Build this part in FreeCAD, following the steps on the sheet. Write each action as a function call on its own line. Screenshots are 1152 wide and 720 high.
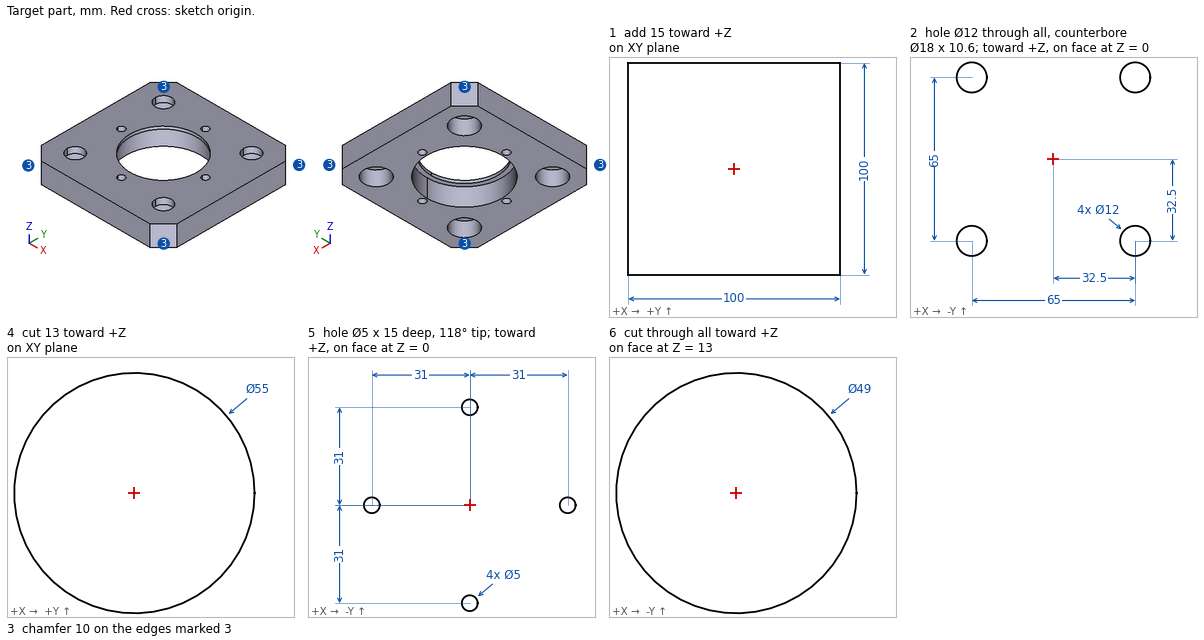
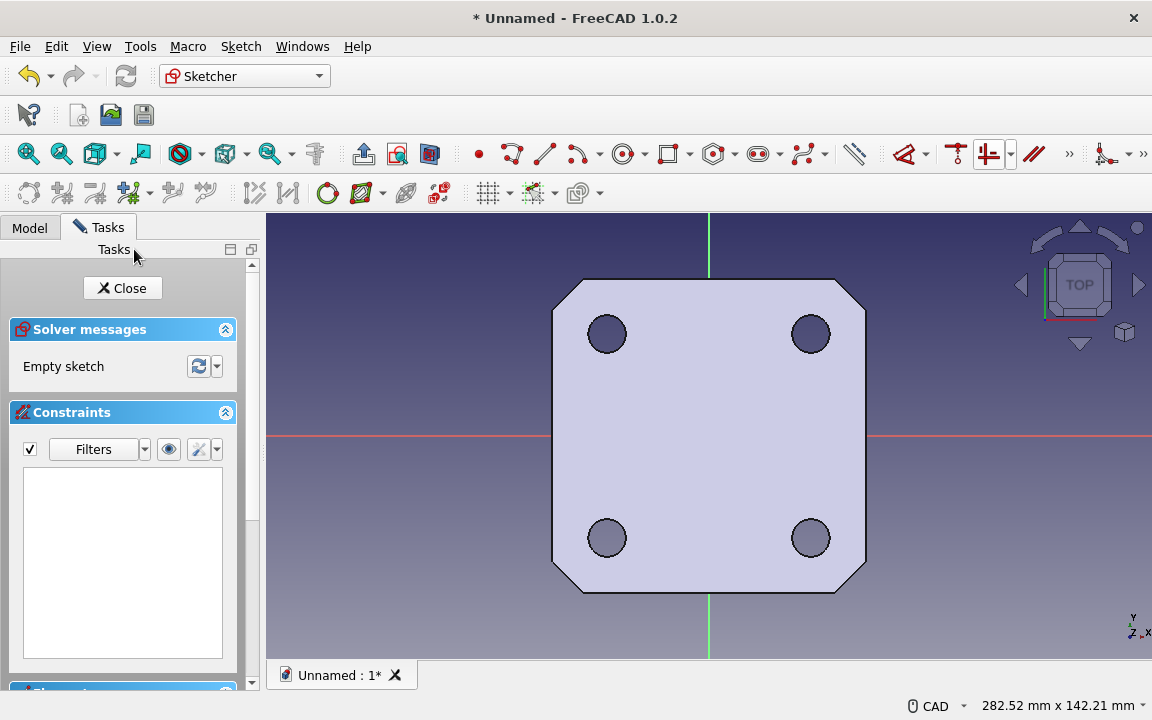
click(430, 154)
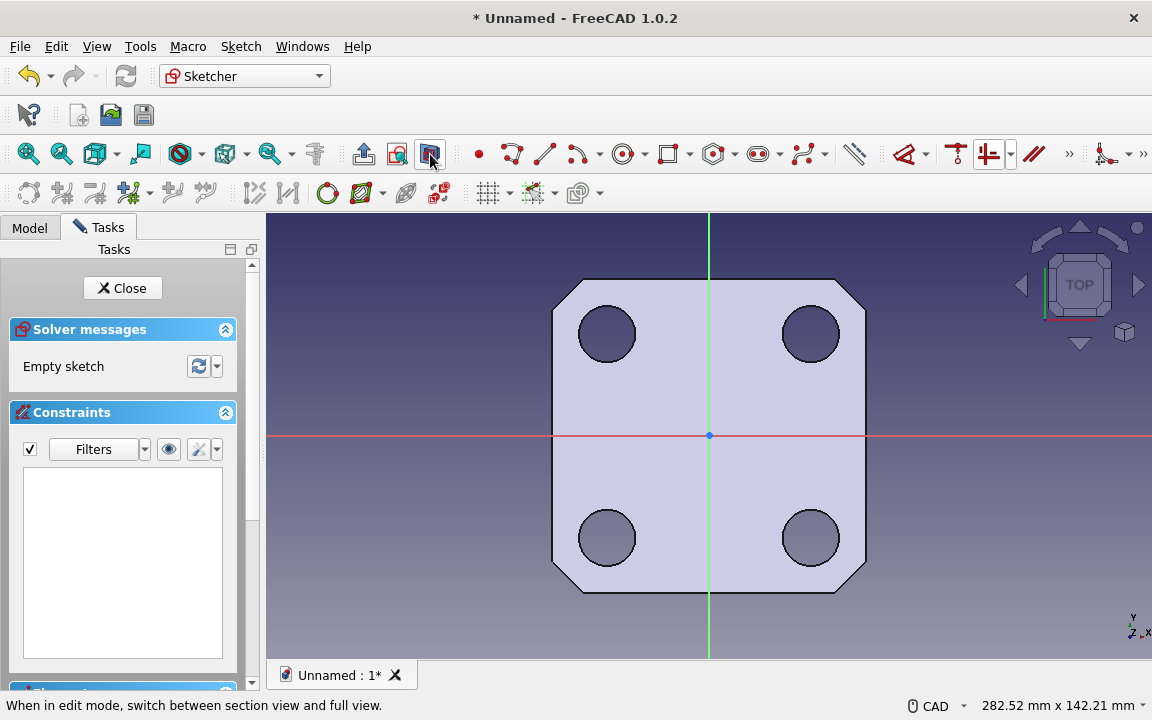
scroll(848, 436, up, 2)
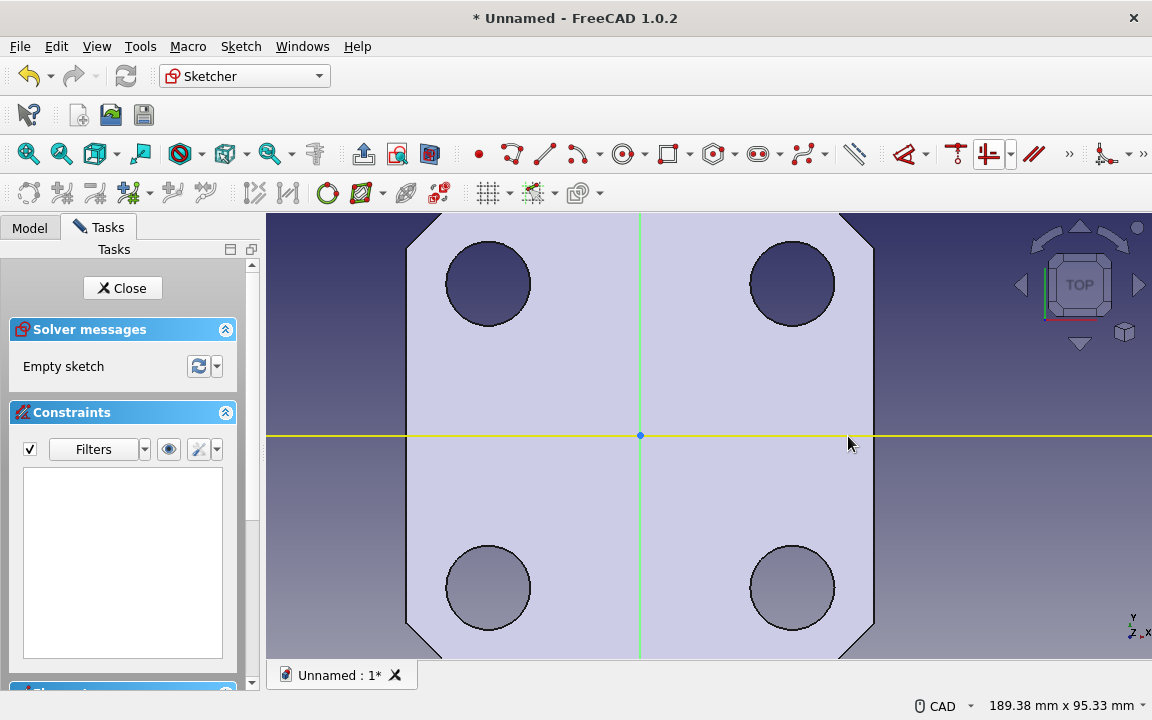
click(622, 154)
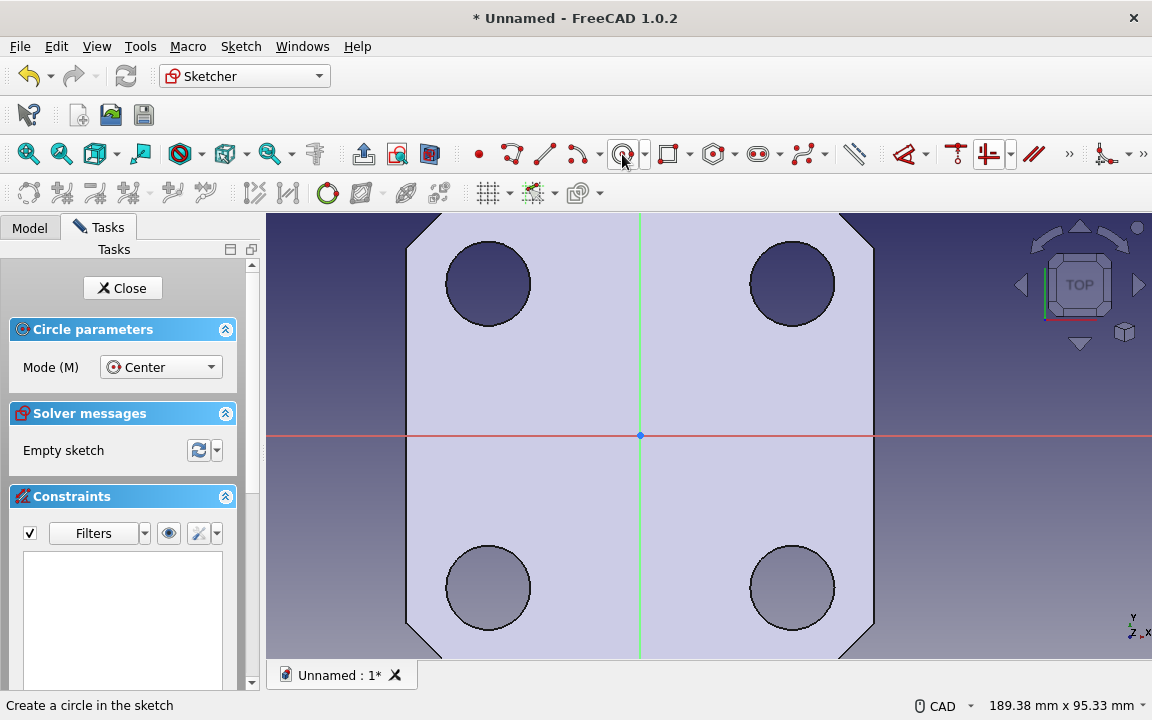
click(640, 436)
move(731, 345)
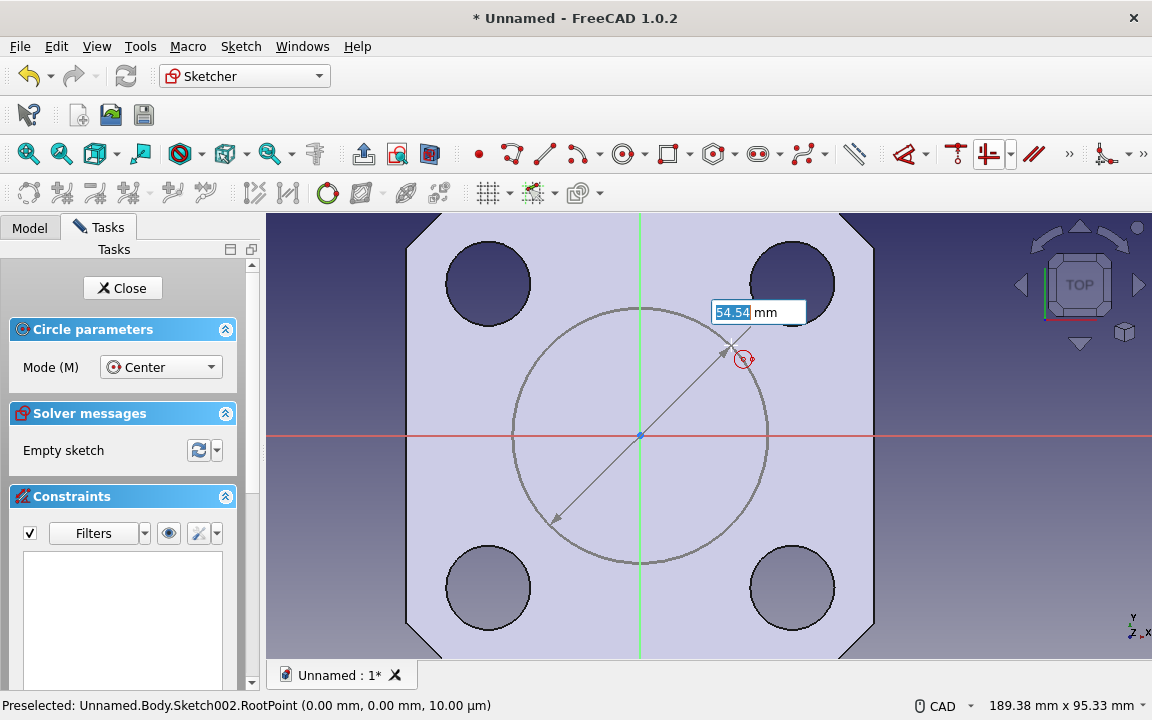
text(55)
key(Return)
key(Escape)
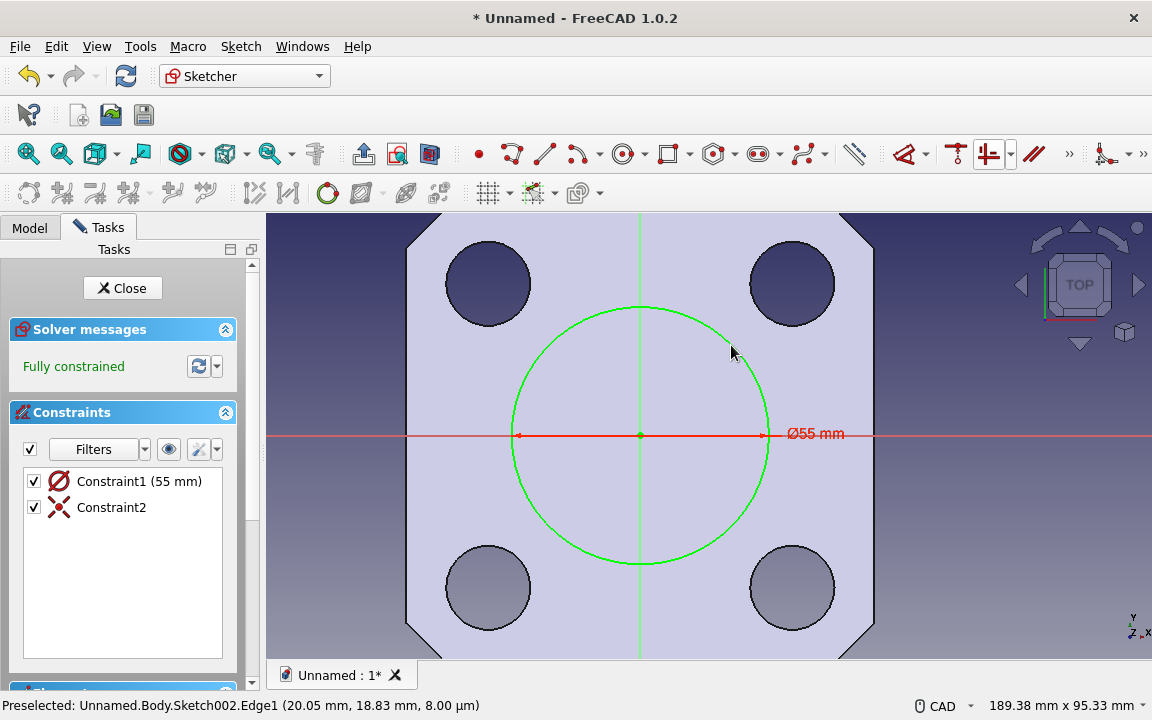
click(123, 288)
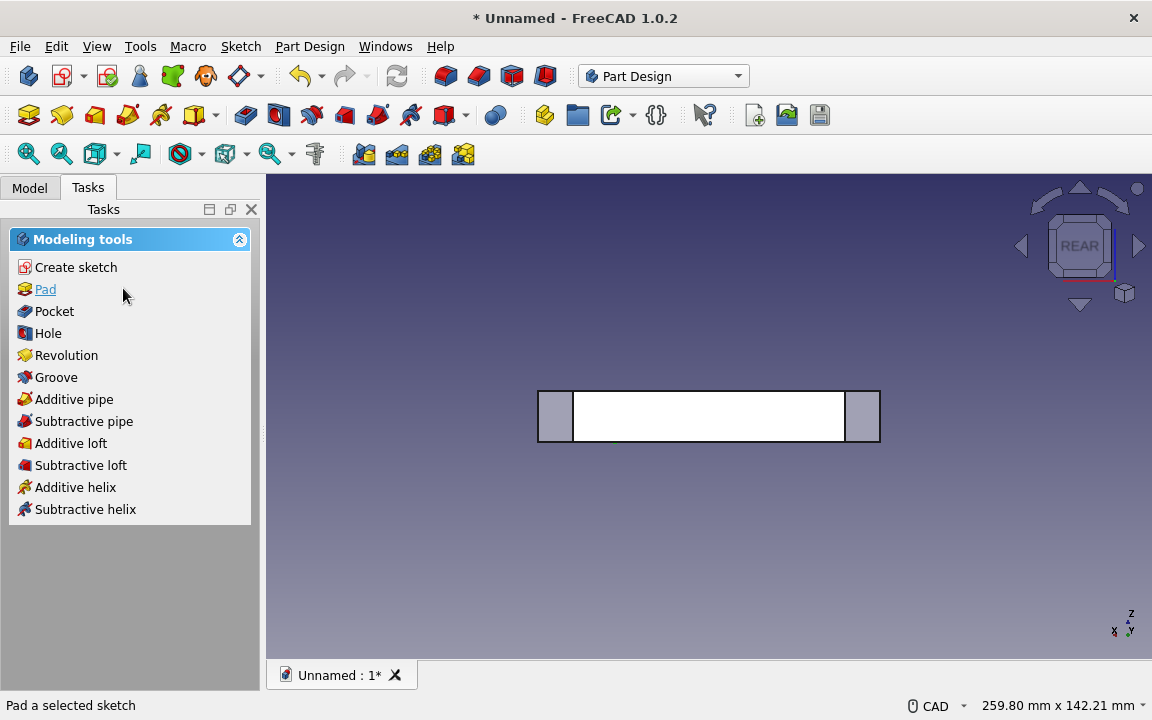
click(246, 116)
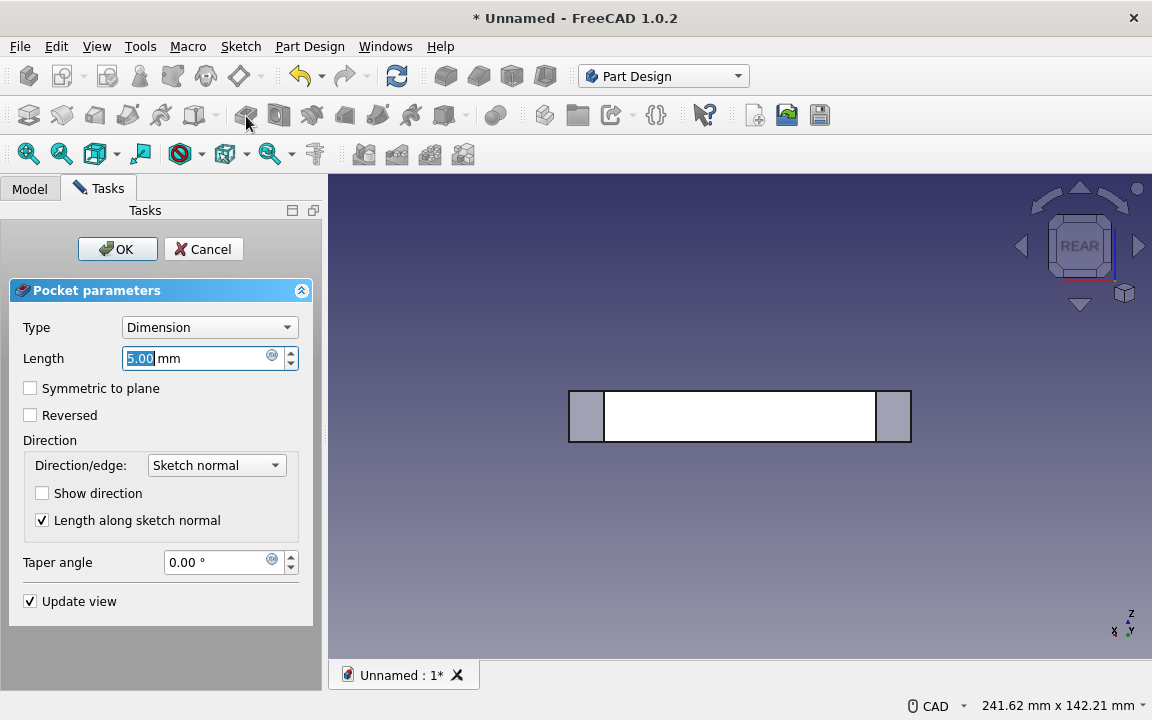
text(13)
key(Tab)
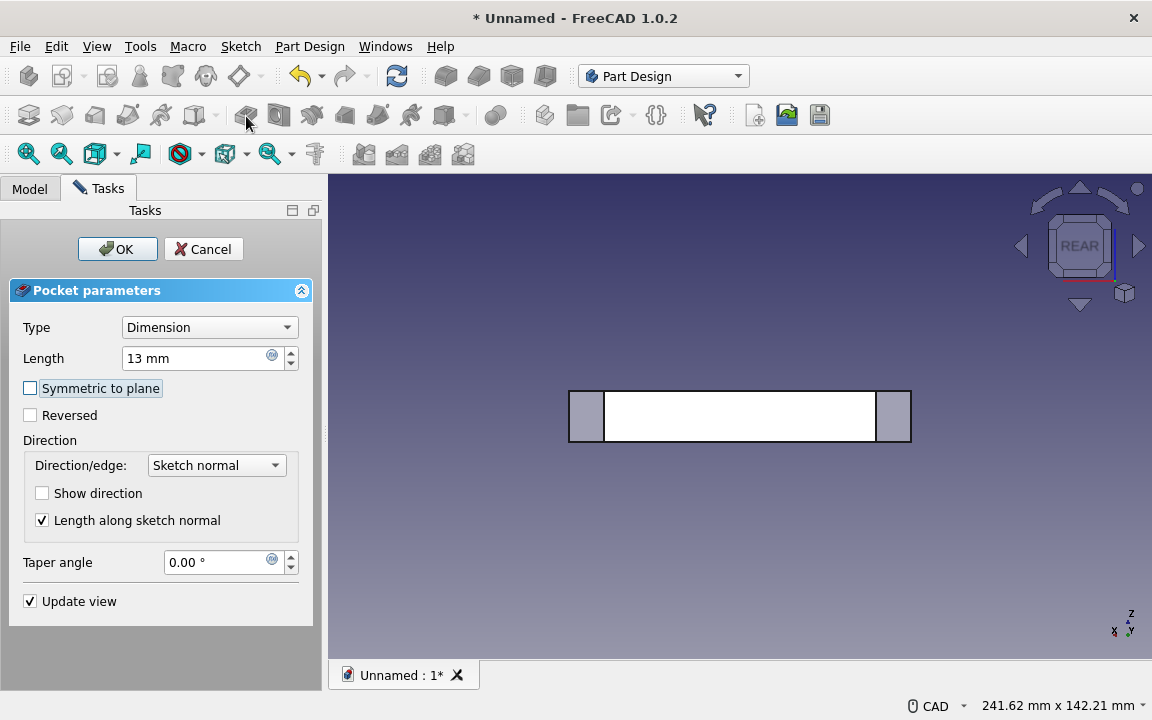
click(31, 415)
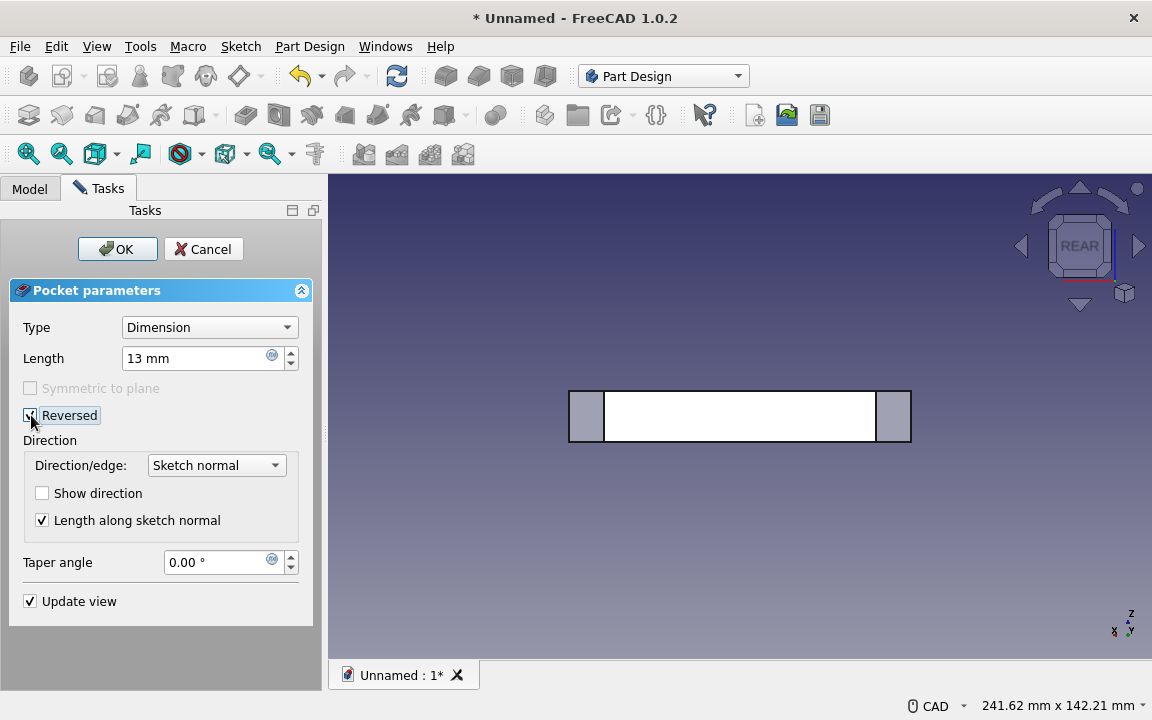
click(118, 249)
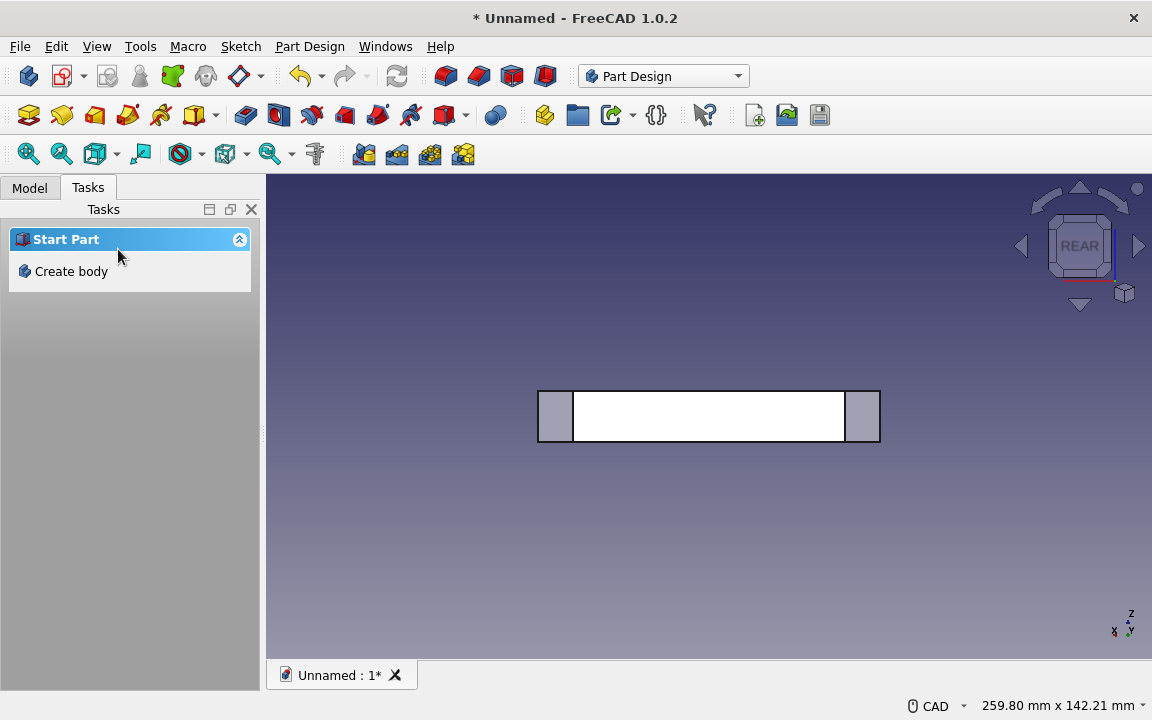
click(29, 154)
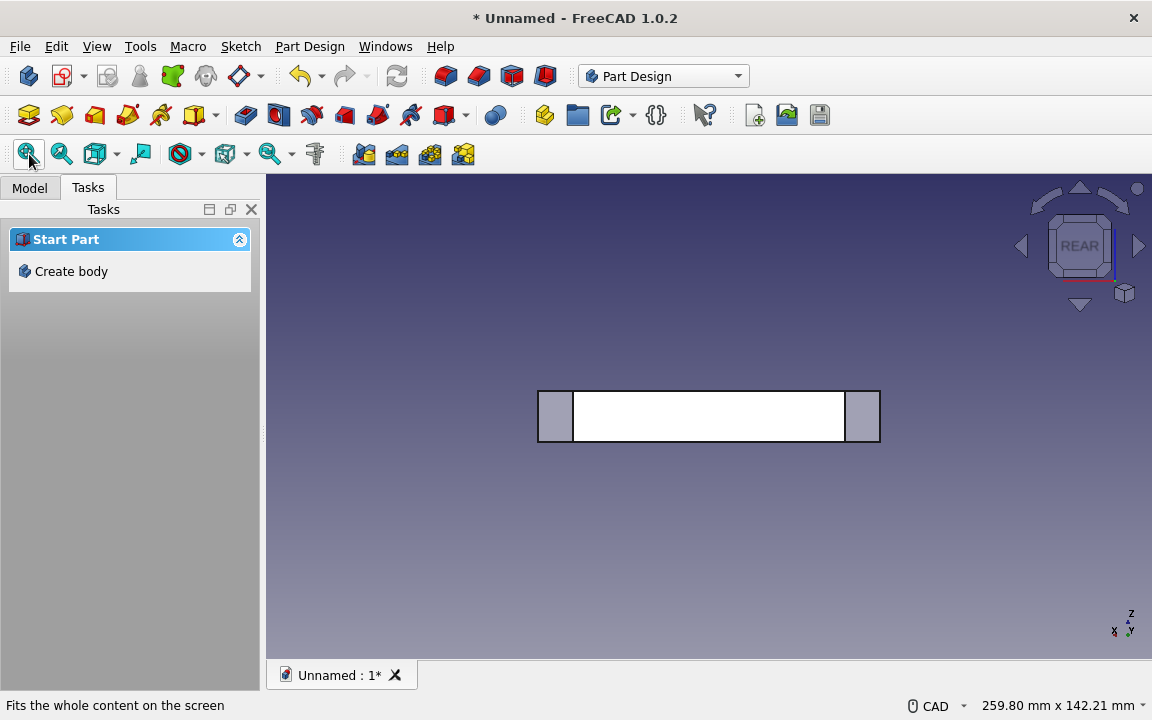
key(5)